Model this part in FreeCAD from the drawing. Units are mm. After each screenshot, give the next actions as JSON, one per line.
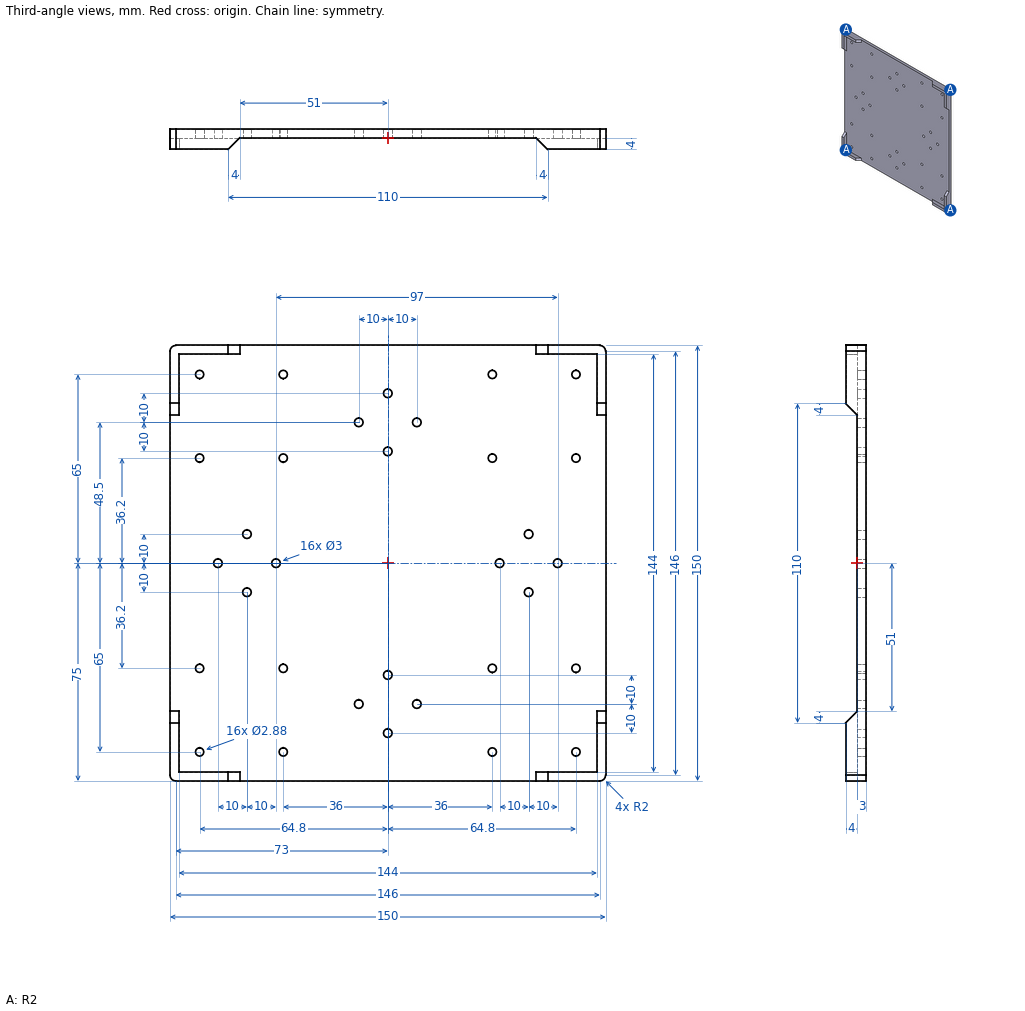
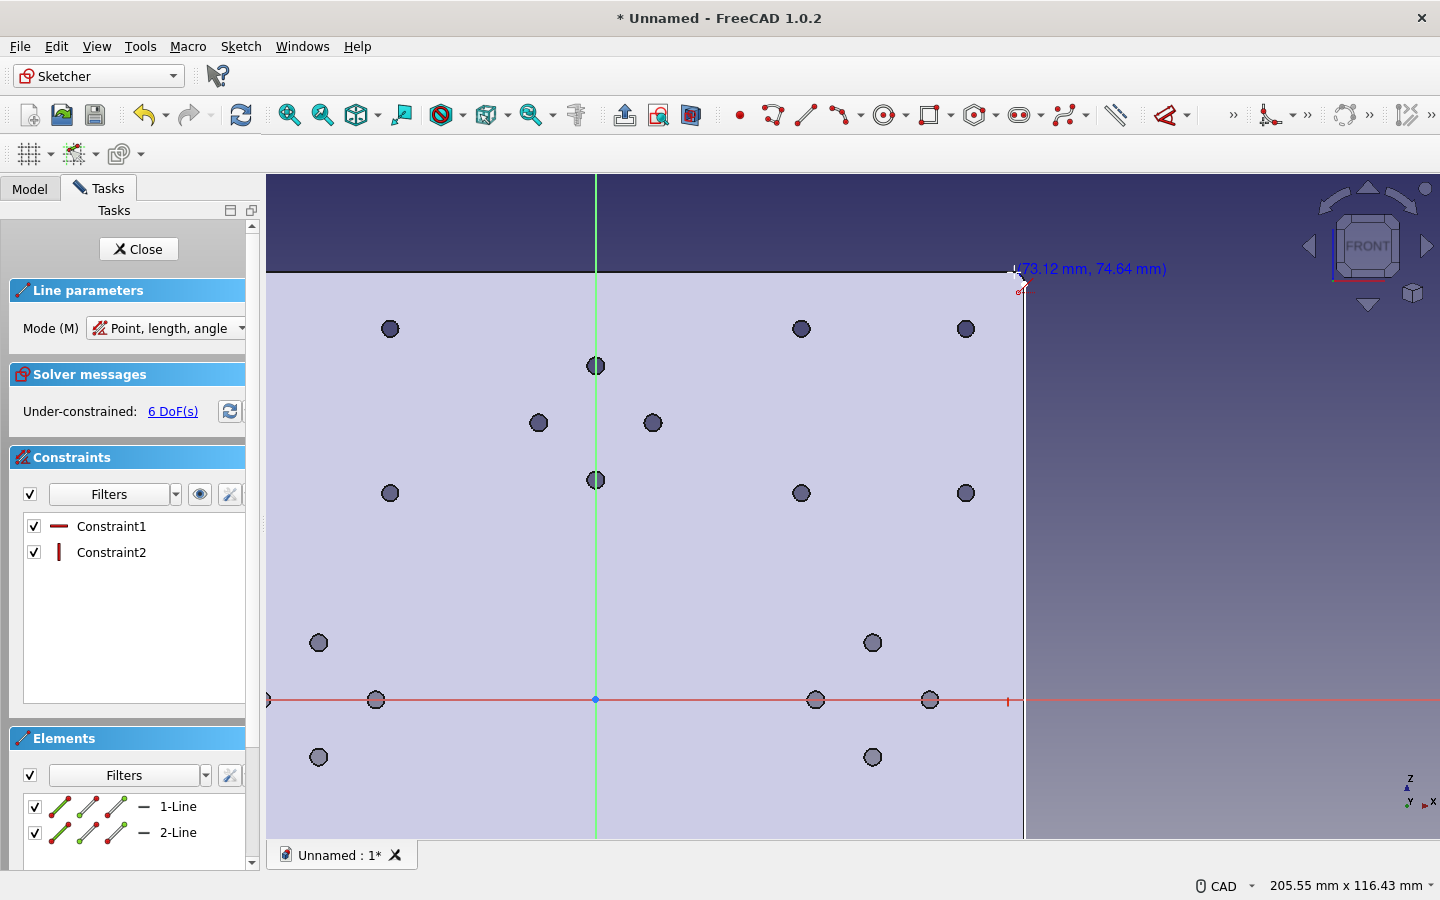
{"action": "left_click", "coordinate": [1013, 272]}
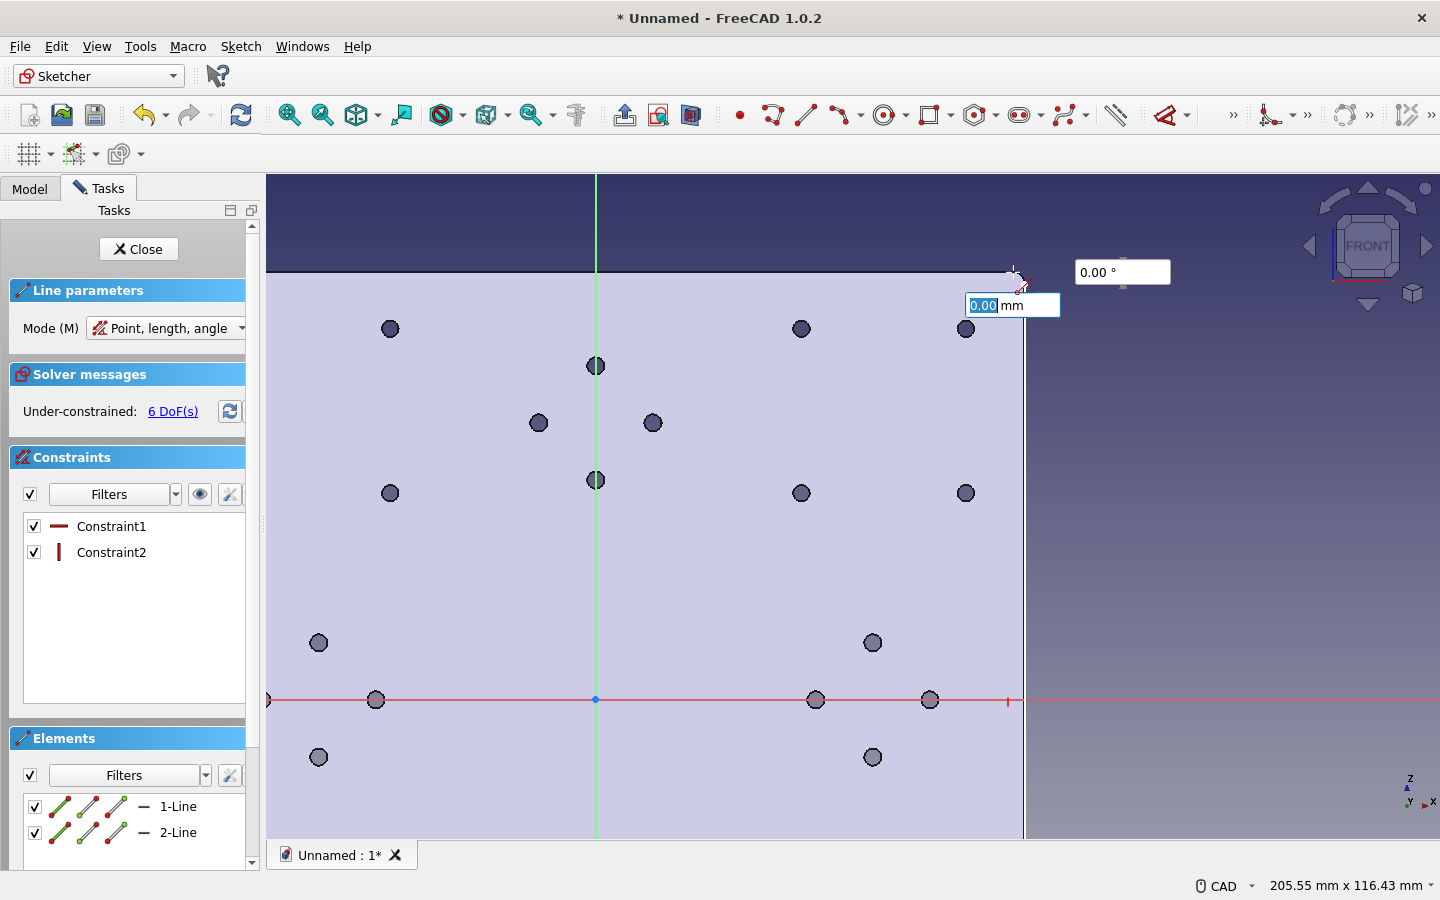
{"action": "scroll", "coordinate": [1014, 271], "scroll_direction": "down", "scroll_amount": 3}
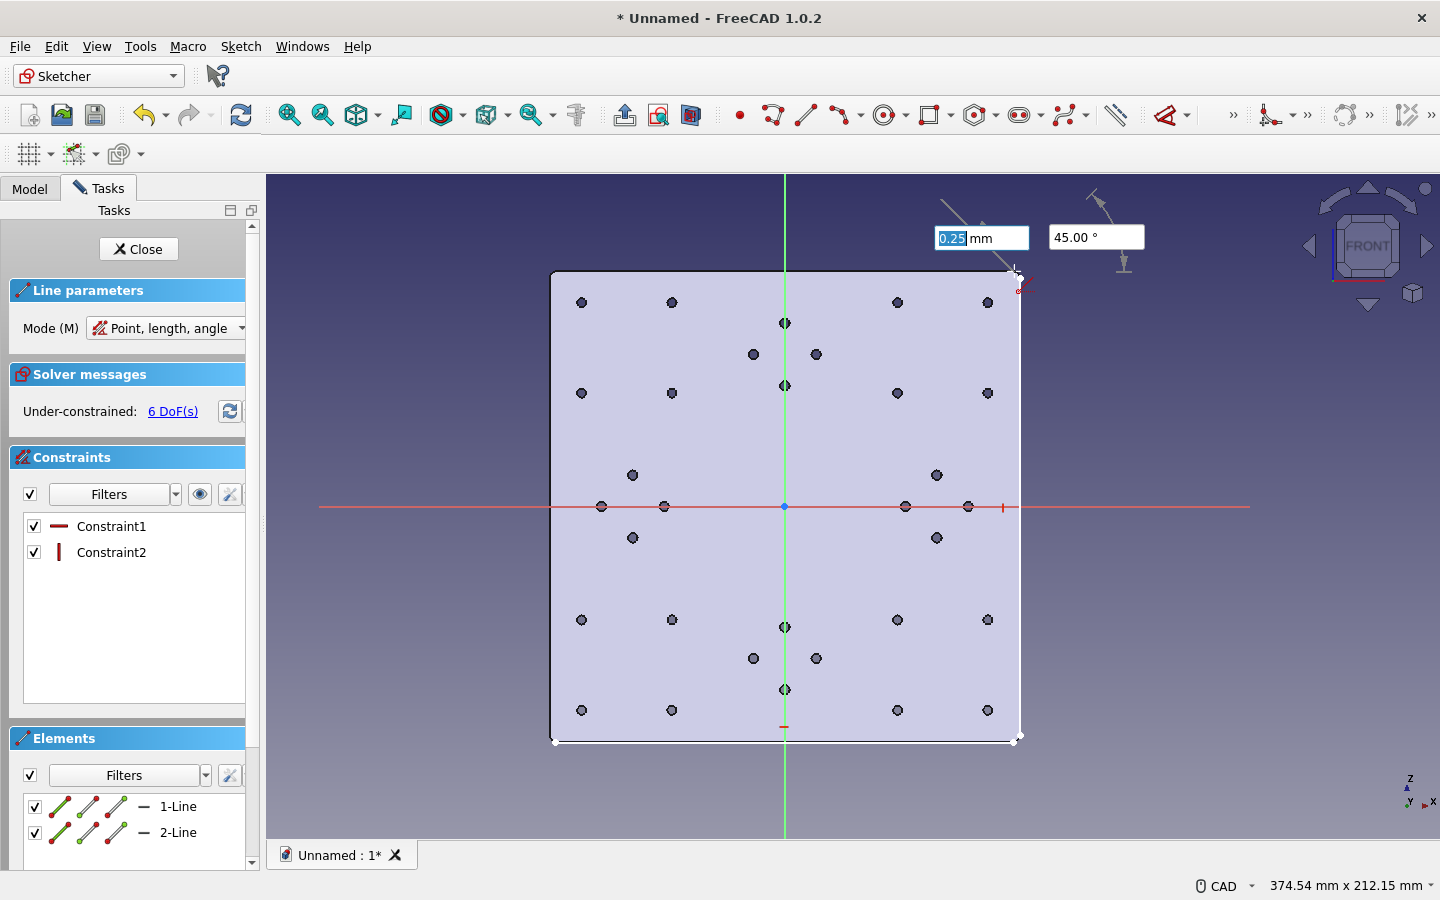
{"action": "left_click", "coordinate": [556, 272]}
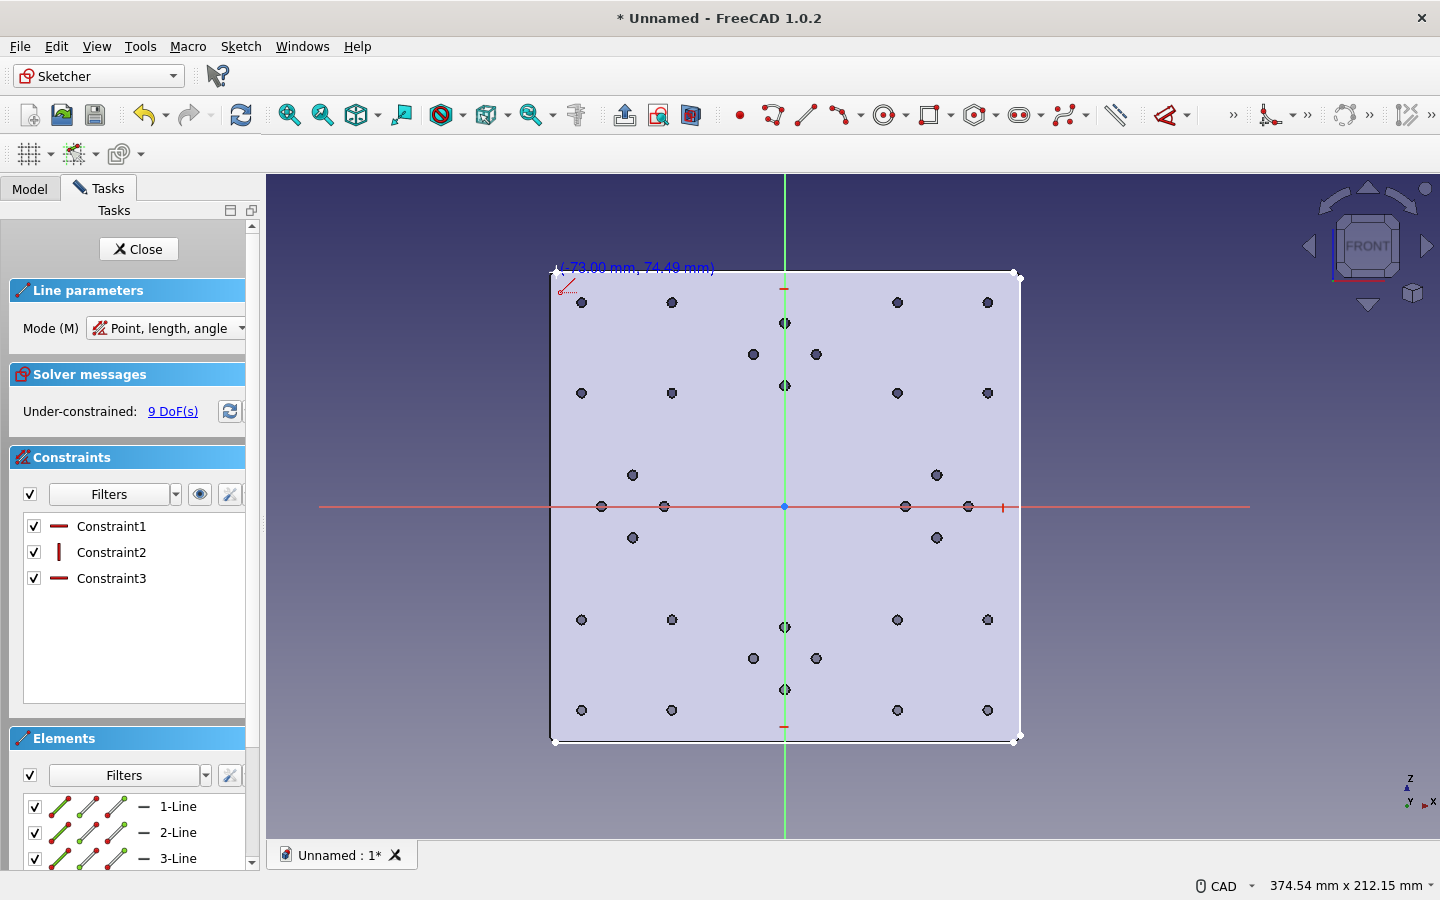
{"action": "scroll", "coordinate": [550, 278], "scroll_direction": "up", "scroll_amount": 3}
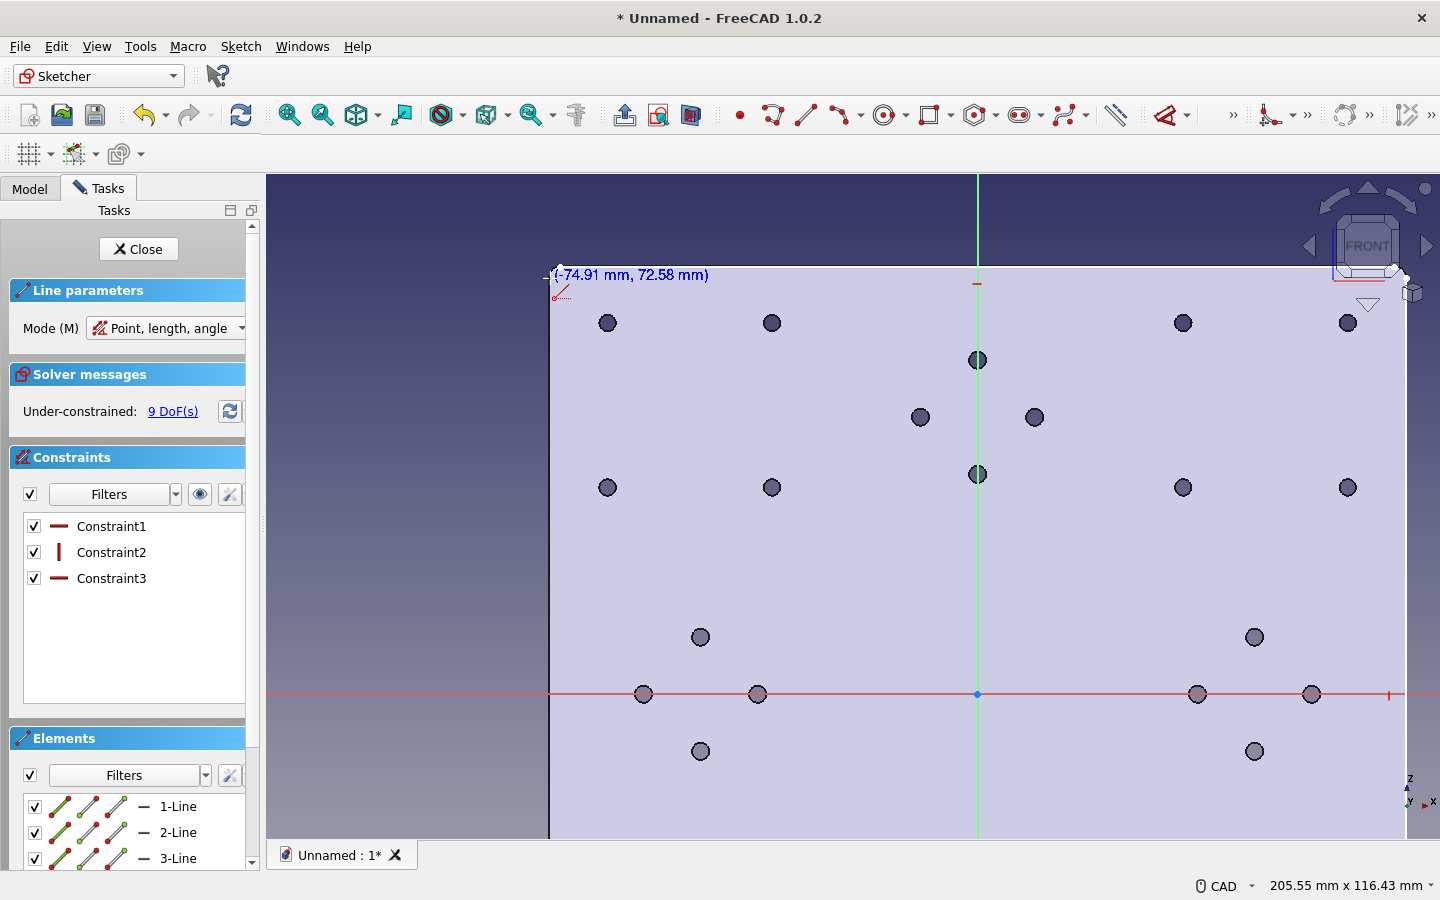
{"action": "left_click", "coordinate": [549, 277]}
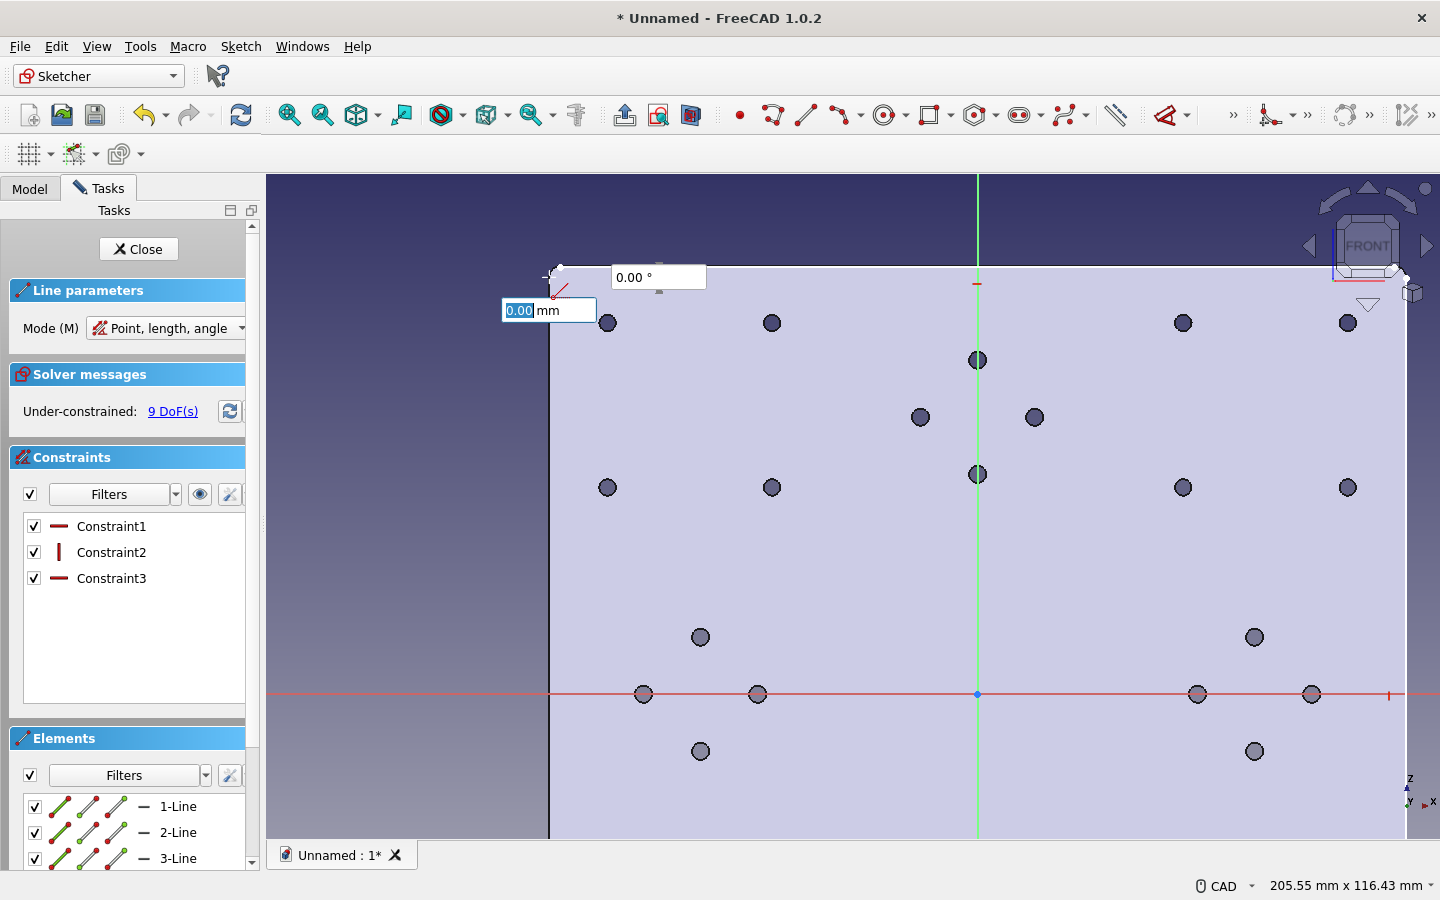
{"action": "scroll", "coordinate": [550, 278], "scroll_direction": "down", "scroll_amount": 3}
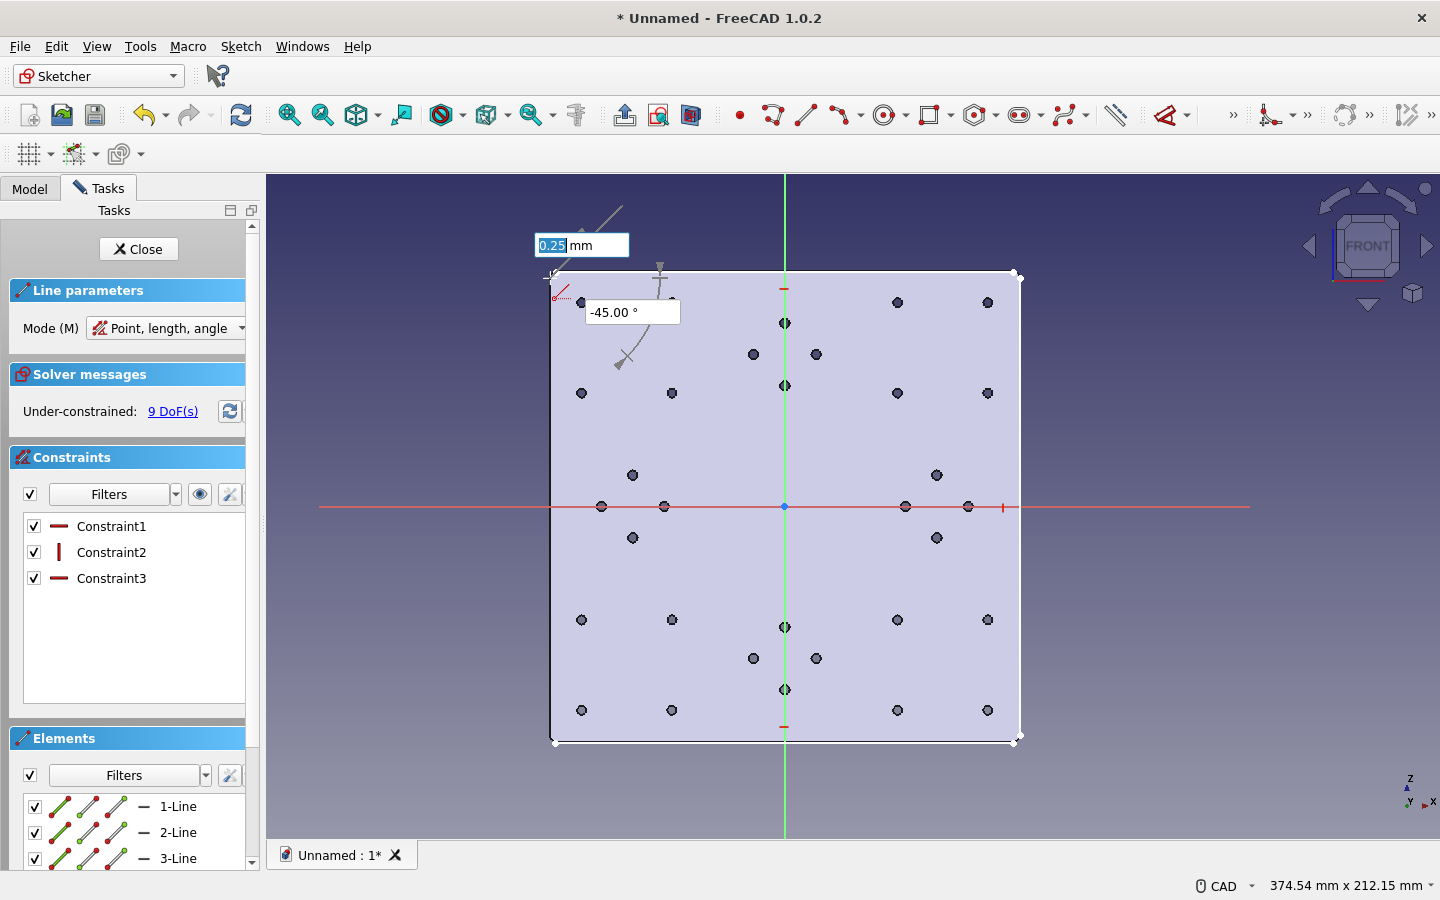
{"action": "scroll", "coordinate": [550, 735], "scroll_direction": "up", "scroll_amount": 3}